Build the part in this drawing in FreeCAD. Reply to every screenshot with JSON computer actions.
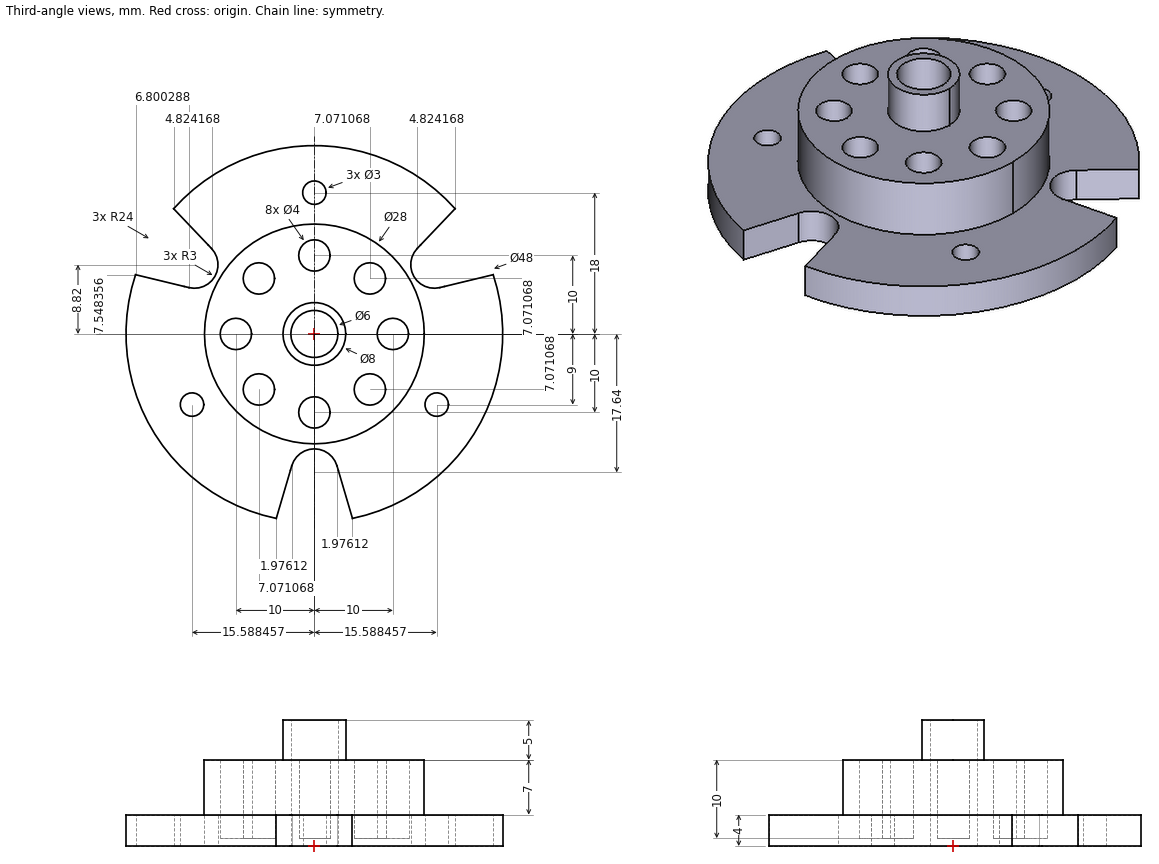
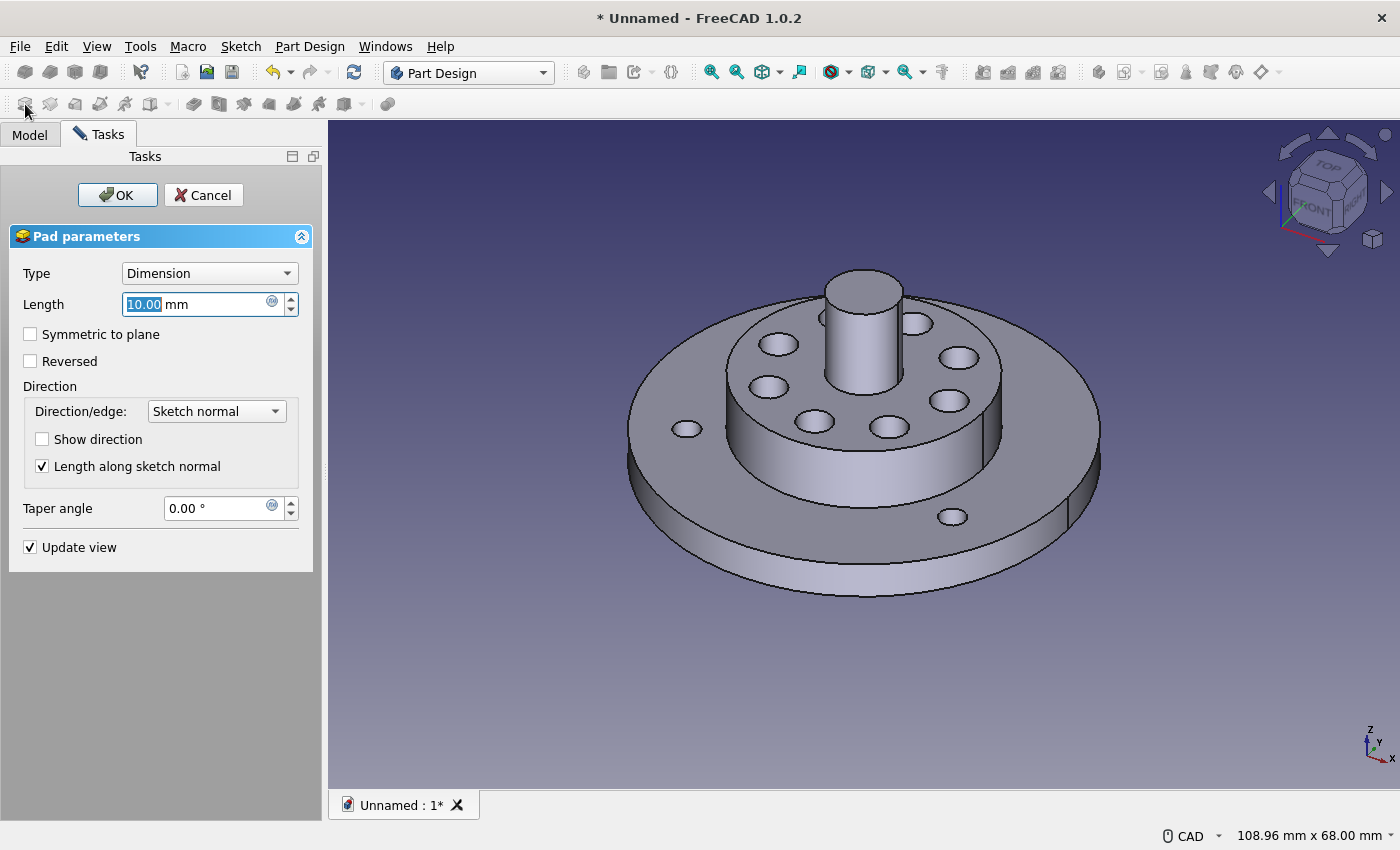
{"action": "type", "text": "5"}
{"action": "key", "text": "Tab"}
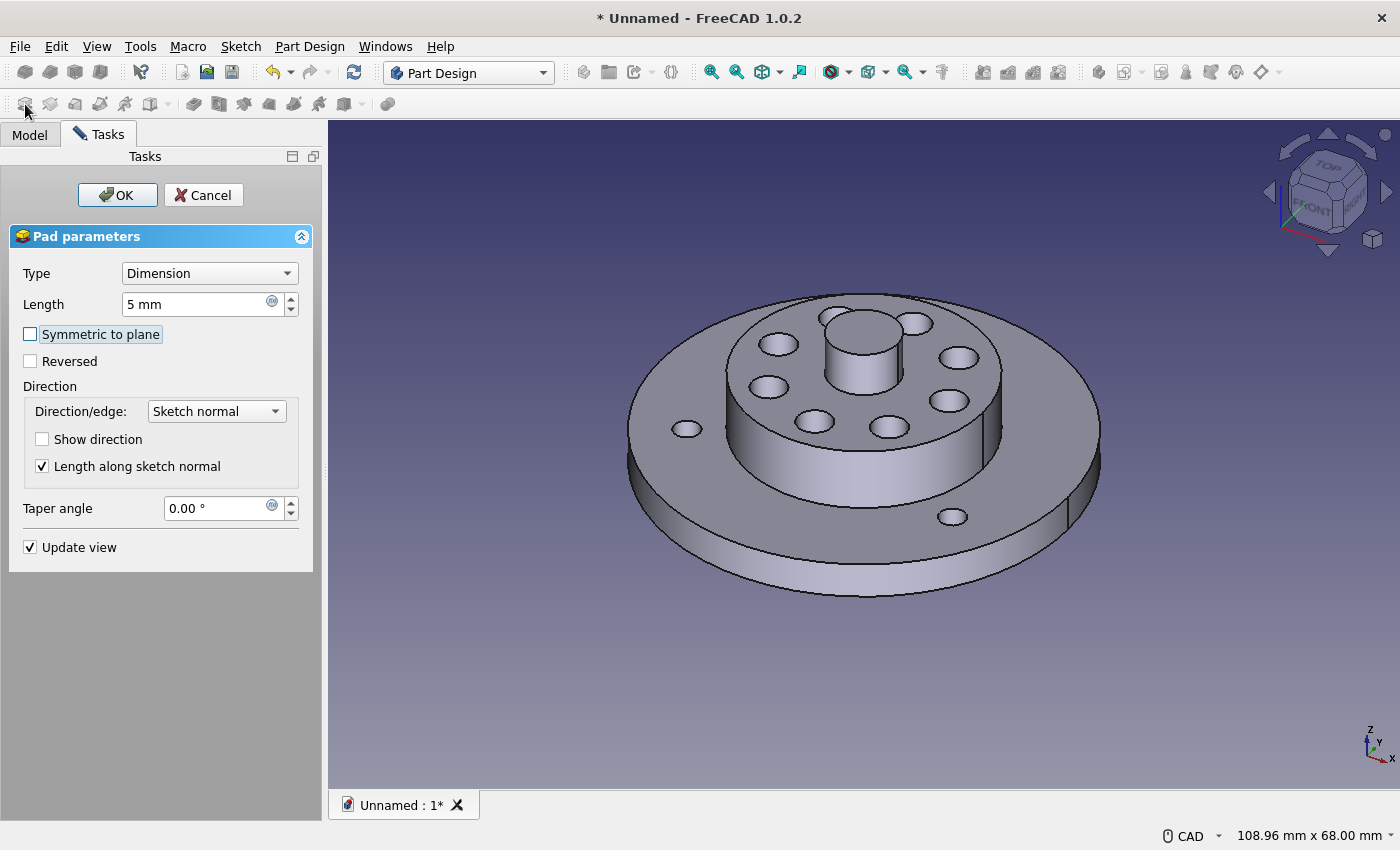
{"action": "left_click", "coordinate": [118, 195]}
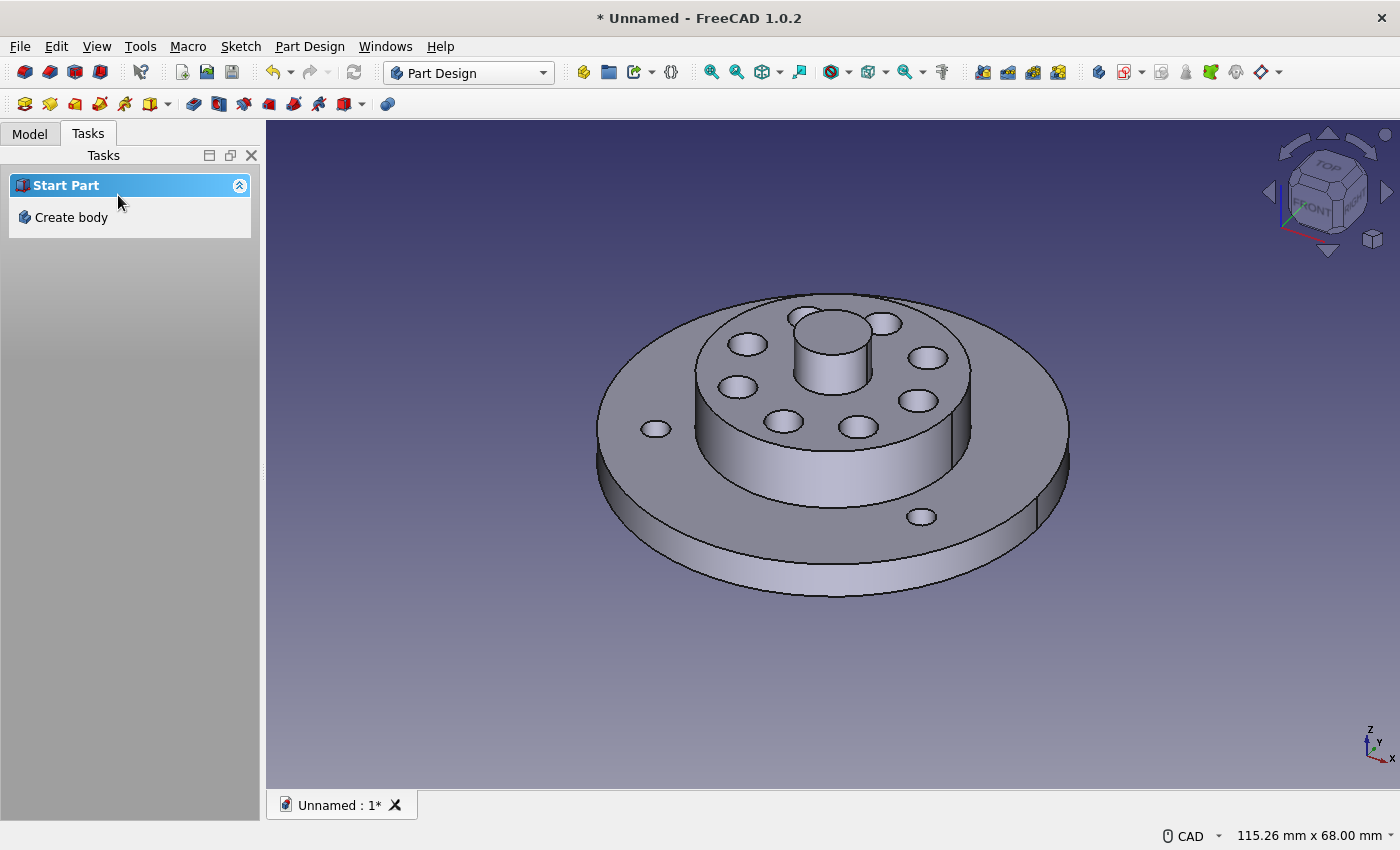
{"action": "left_click", "coordinate": [833, 331]}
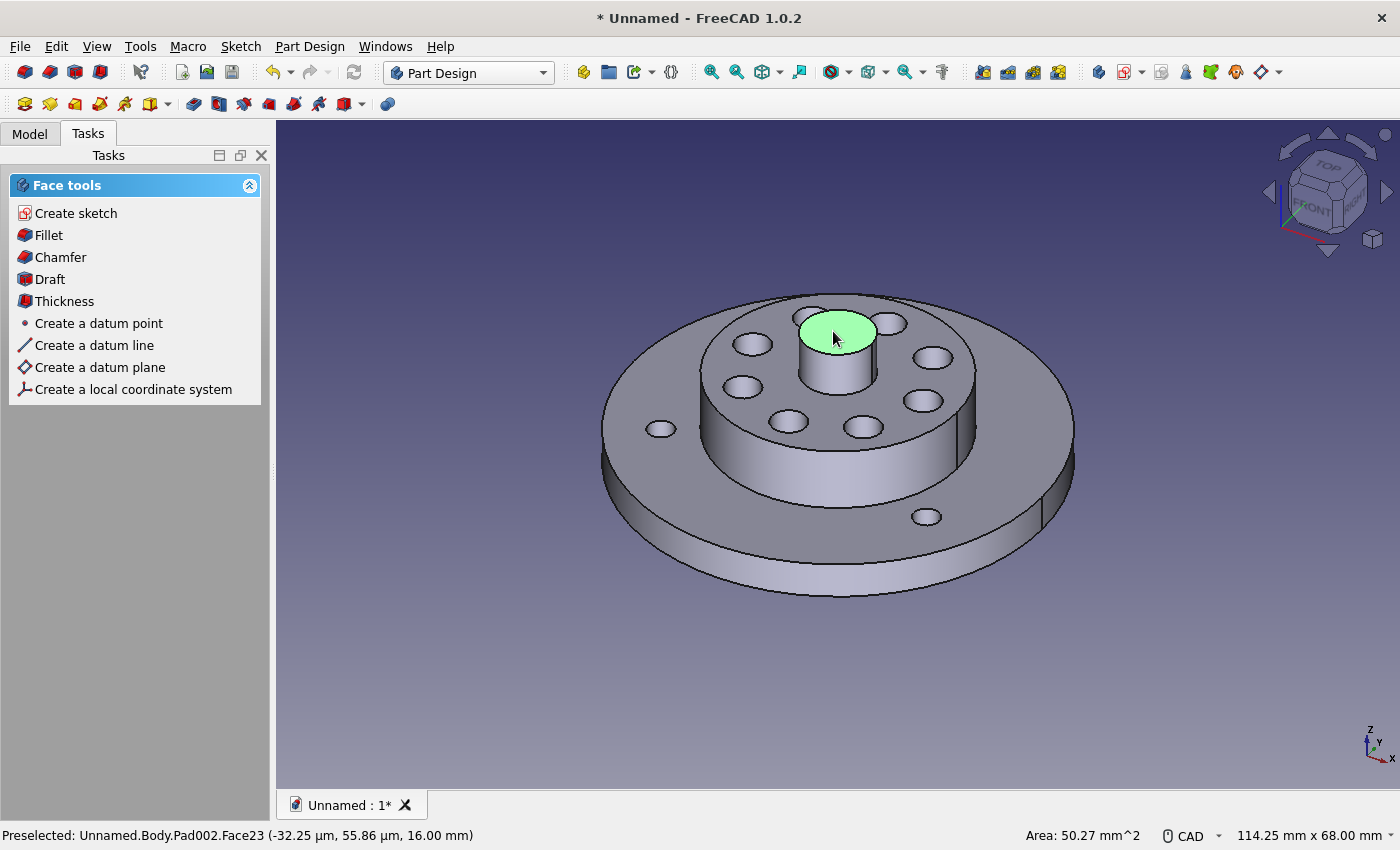
{"action": "left_click", "coordinate": [1124, 72]}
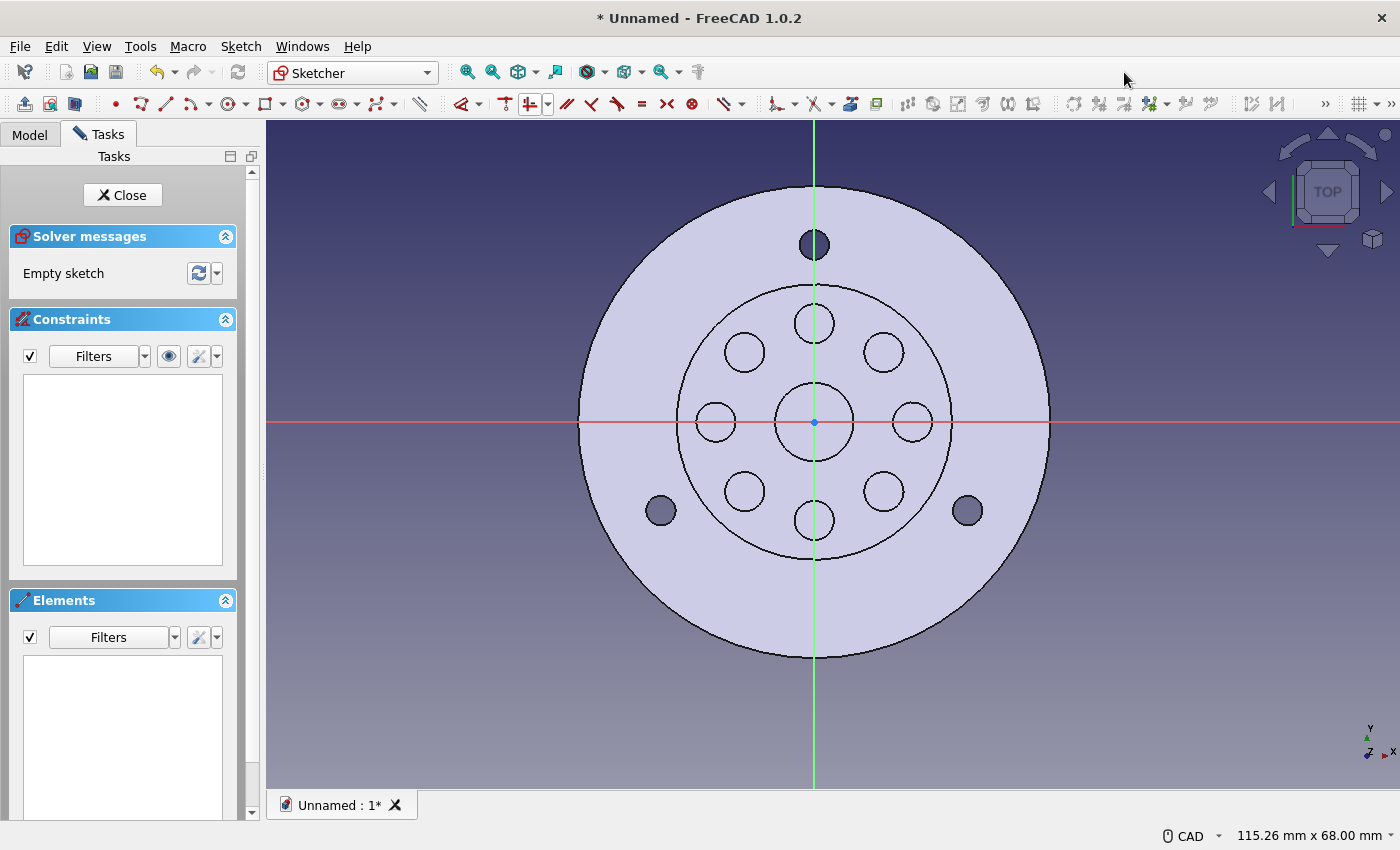
{"action": "scroll", "coordinate": [822, 417], "scroll_direction": "up", "scroll_amount": 10}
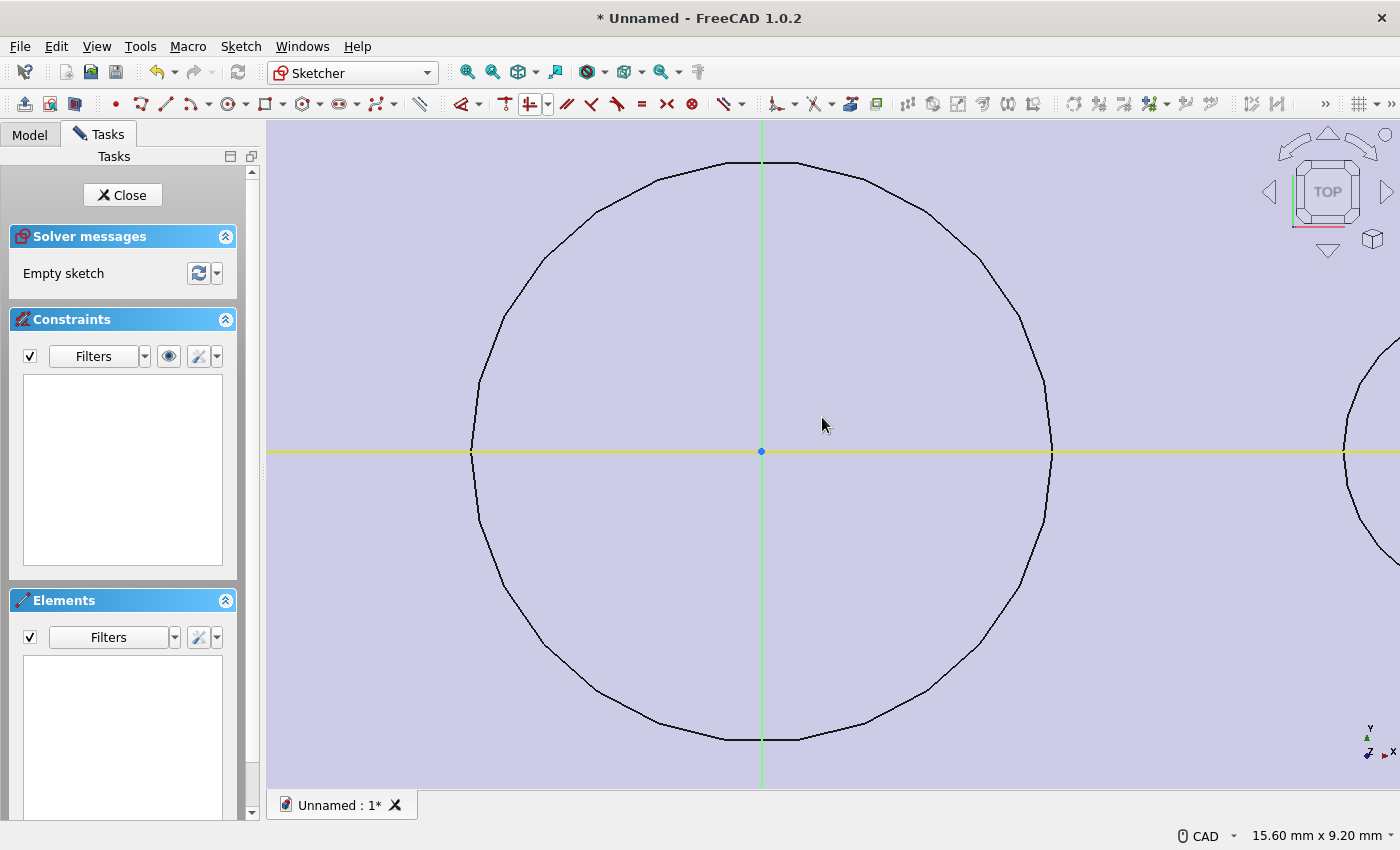
{"action": "left_click", "coordinate": [228, 104]}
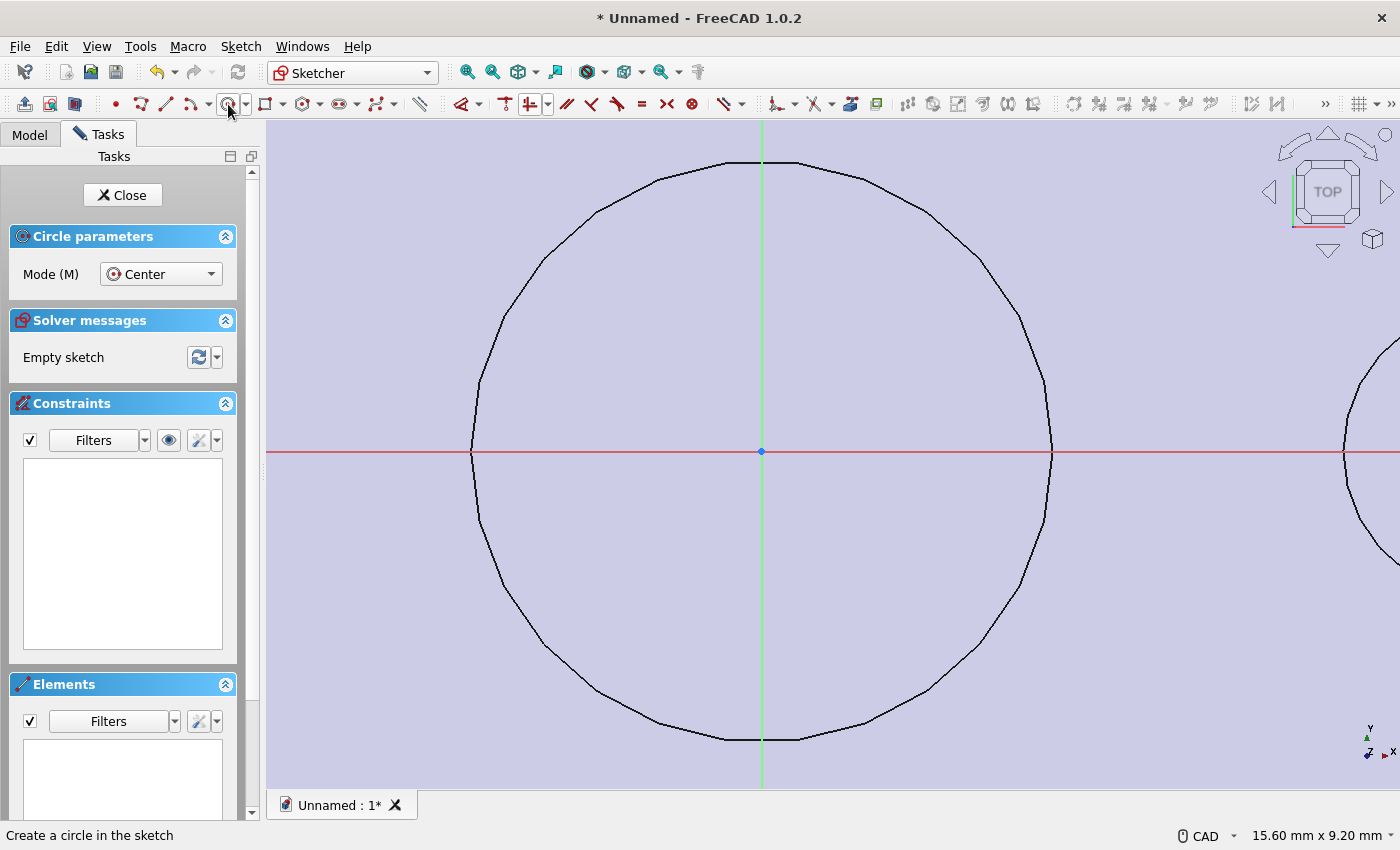
{"action": "left_click", "coordinate": [762, 452]}
{"action": "mouse_move", "coordinate": [916, 297]}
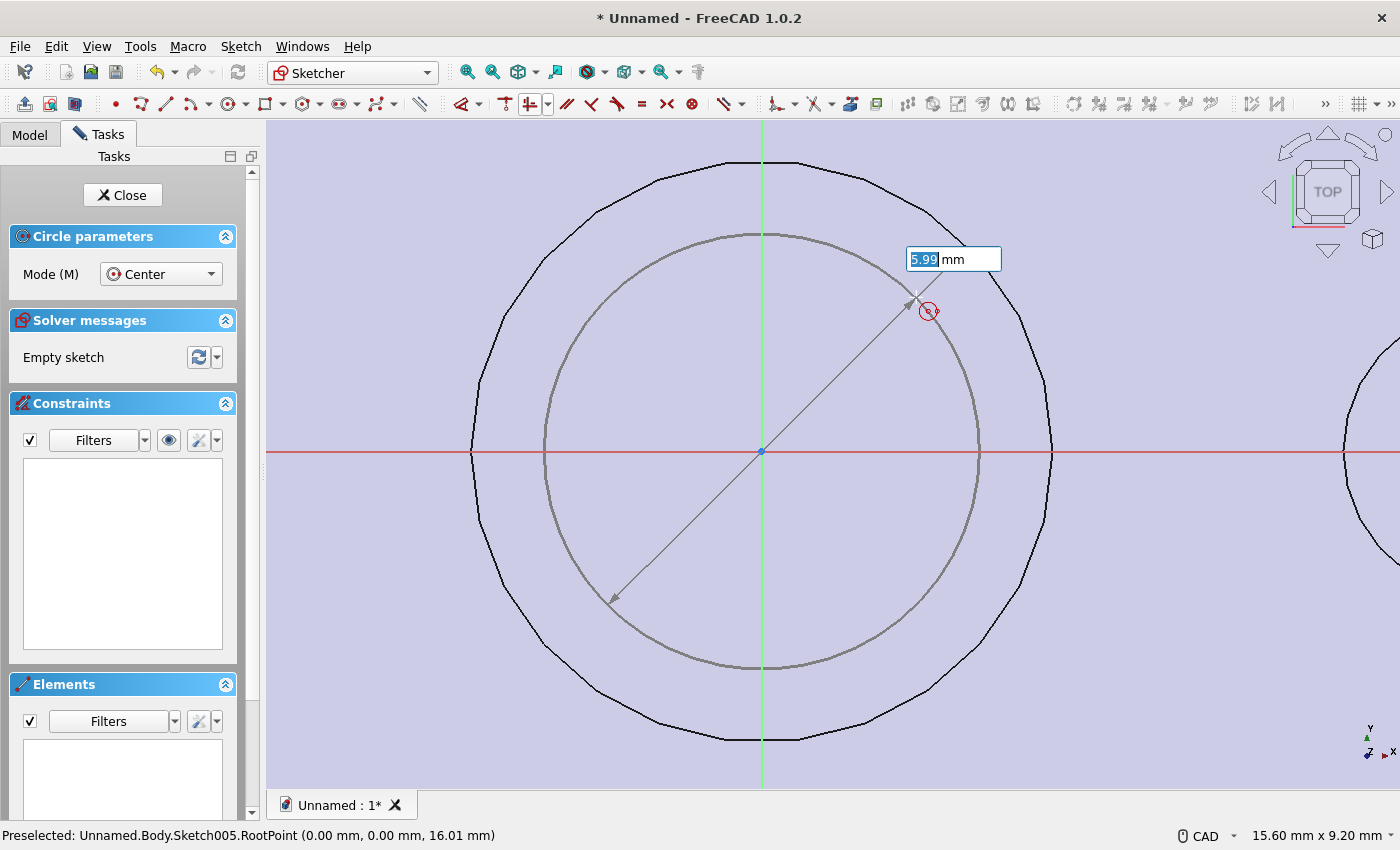
{"action": "type", "text": "6"}
{"action": "key", "text": "Return"}
{"action": "key", "text": "Escape"}